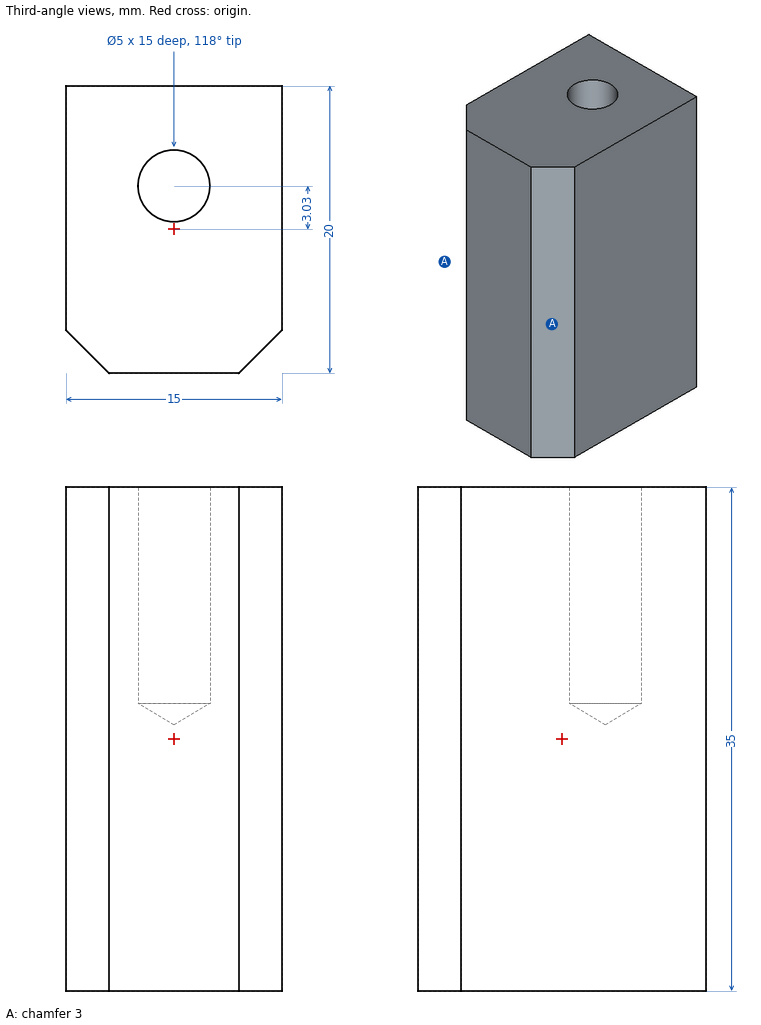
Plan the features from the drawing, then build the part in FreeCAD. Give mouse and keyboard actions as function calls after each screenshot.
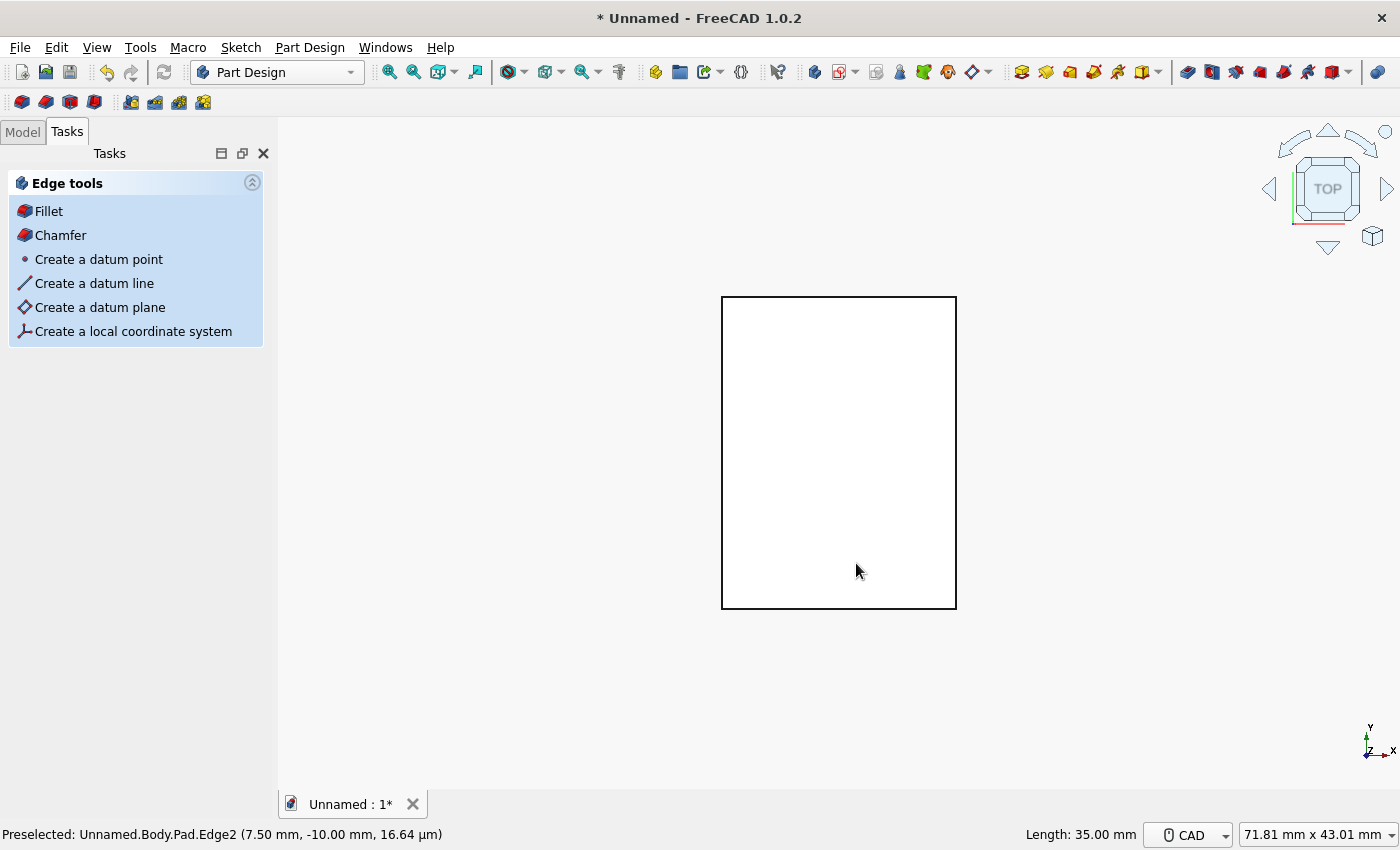
key(1)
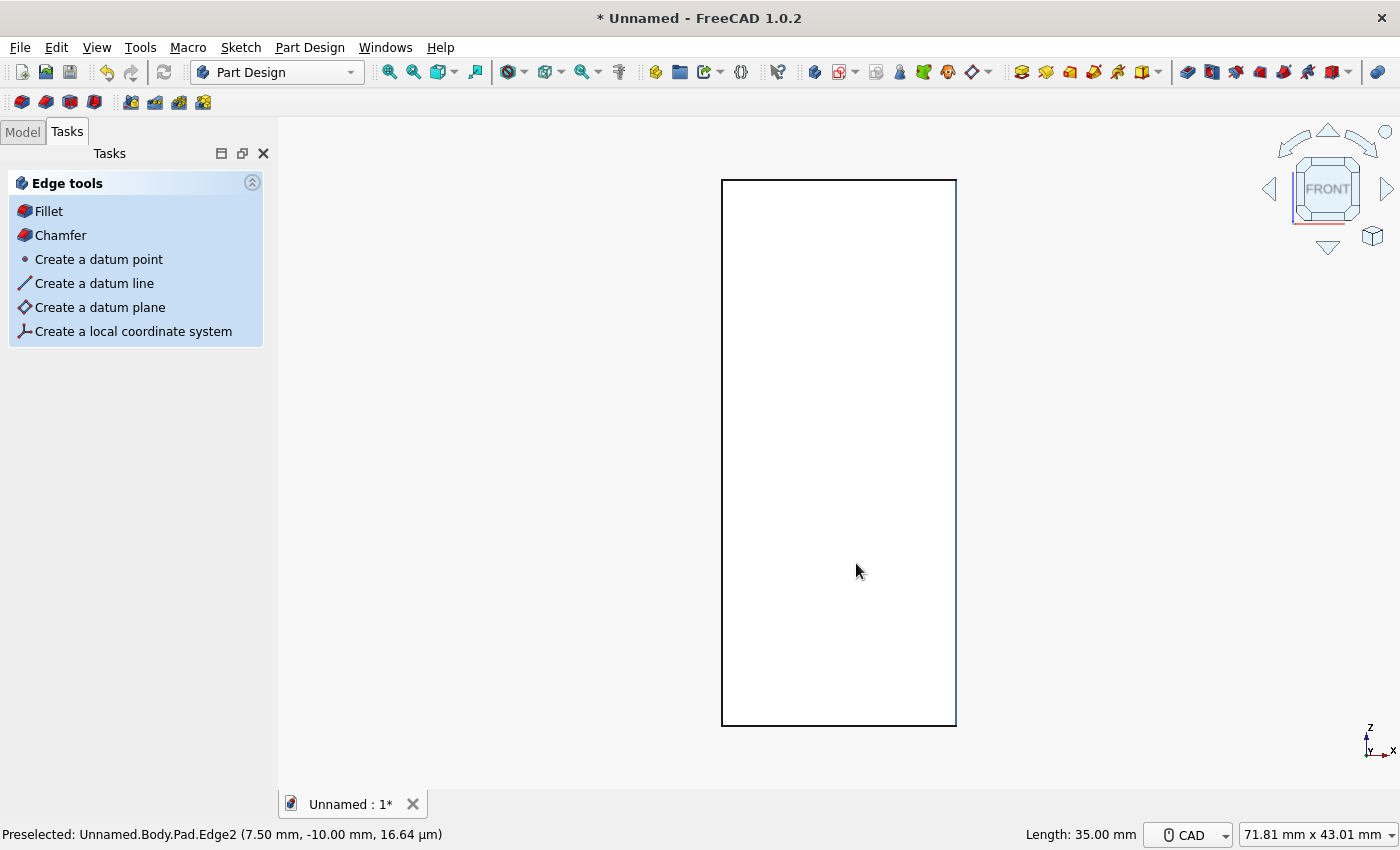
click(722, 452, ctrl)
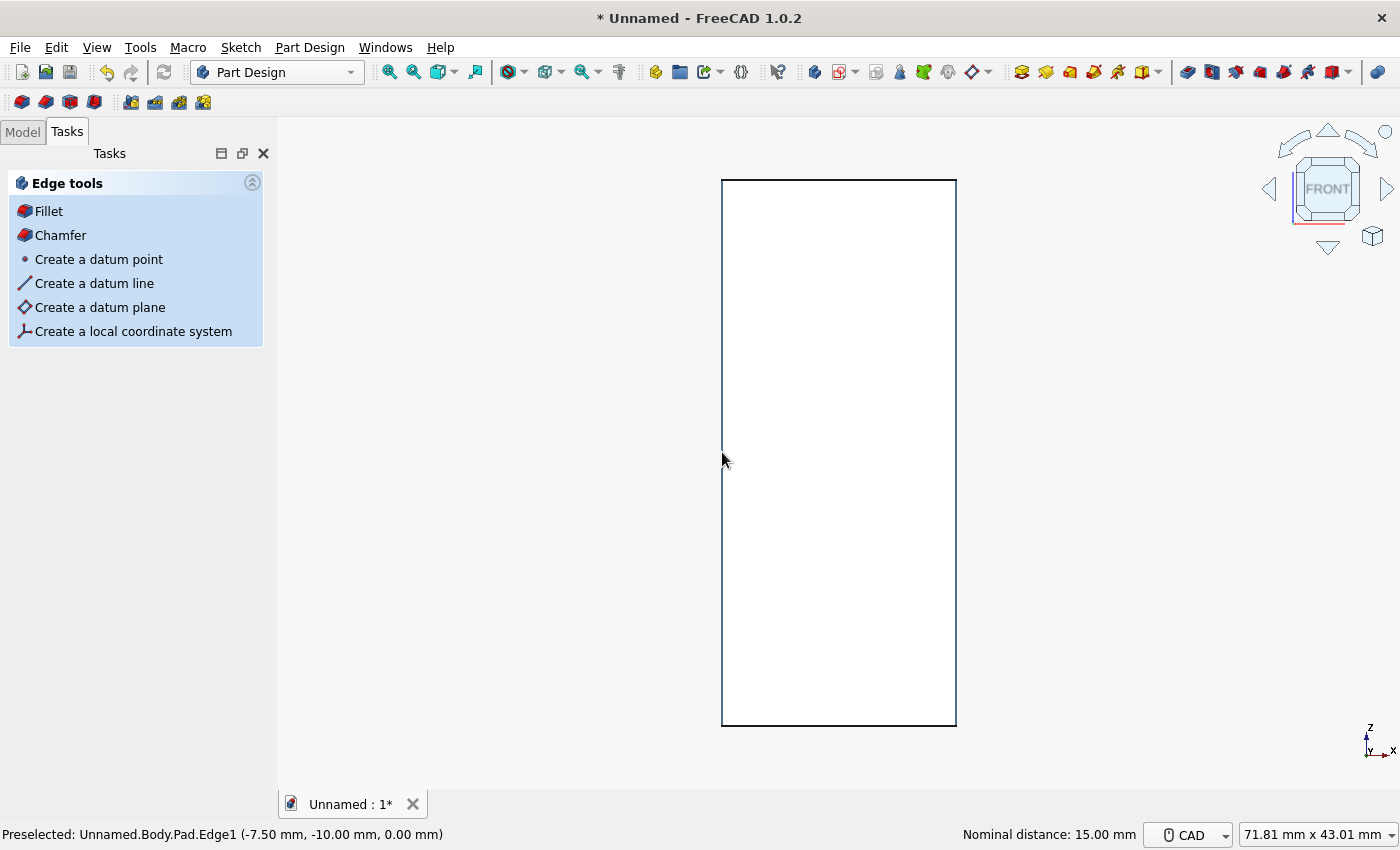
click(46, 102)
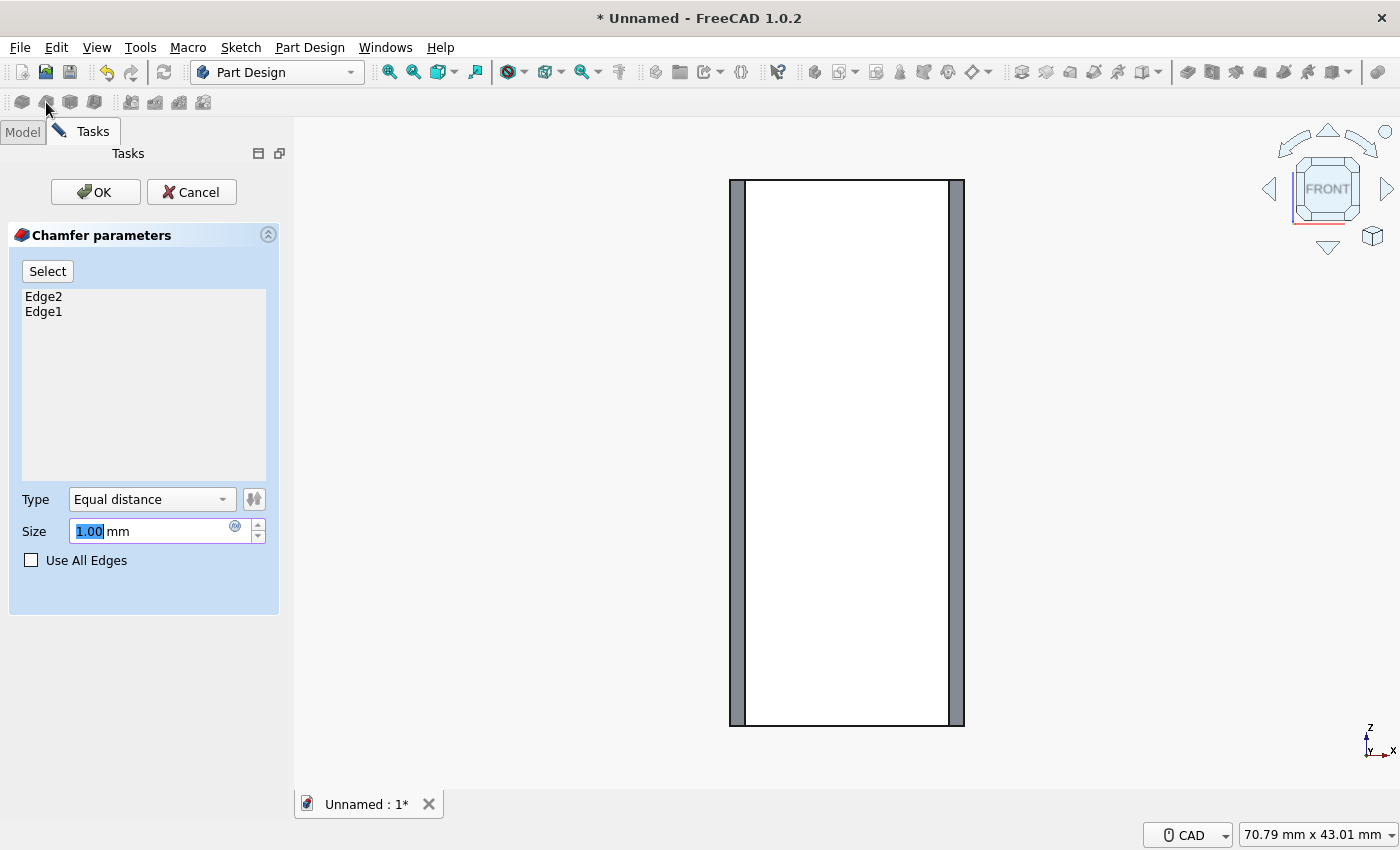
text(3)
key(Tab)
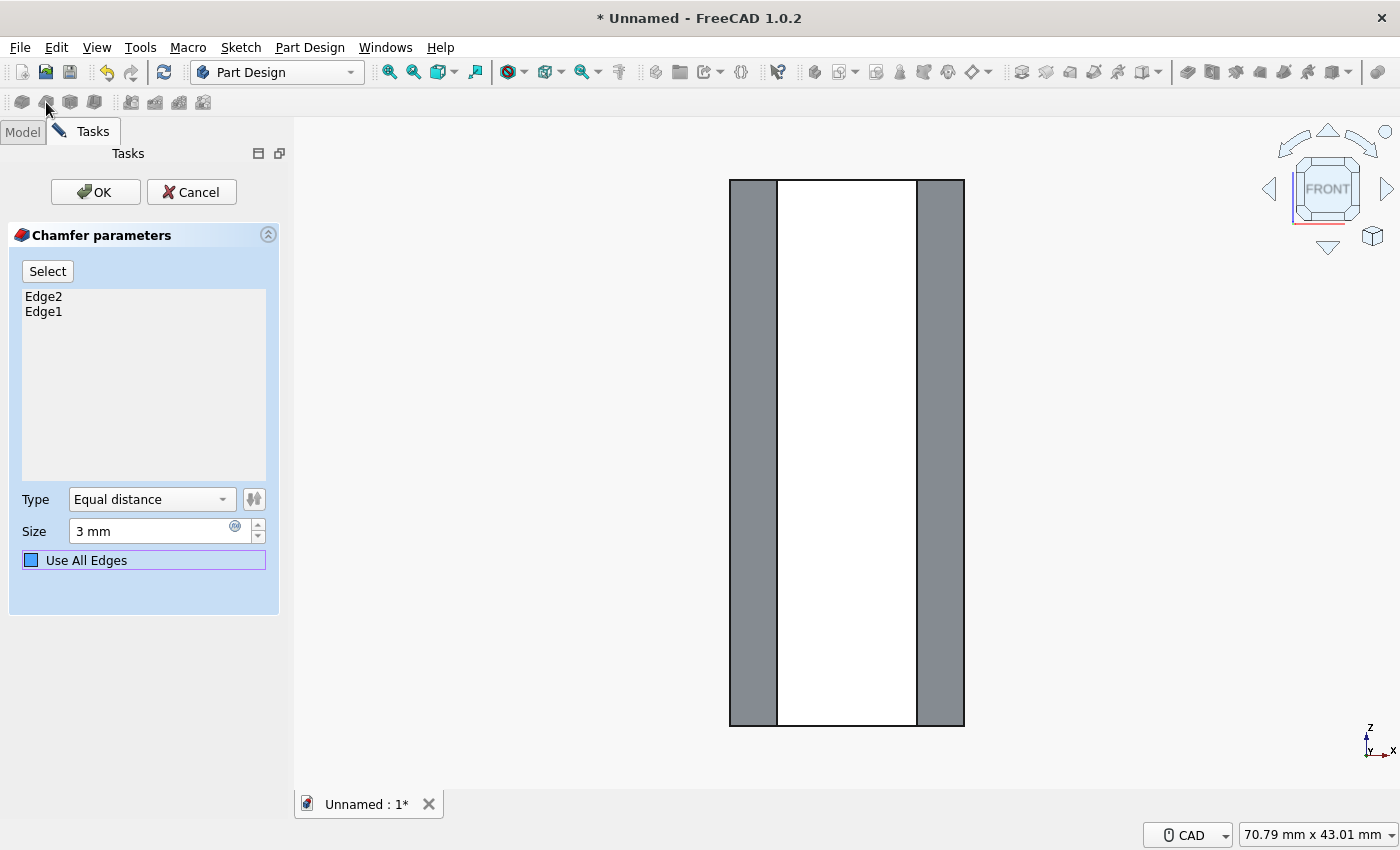
click(96, 192)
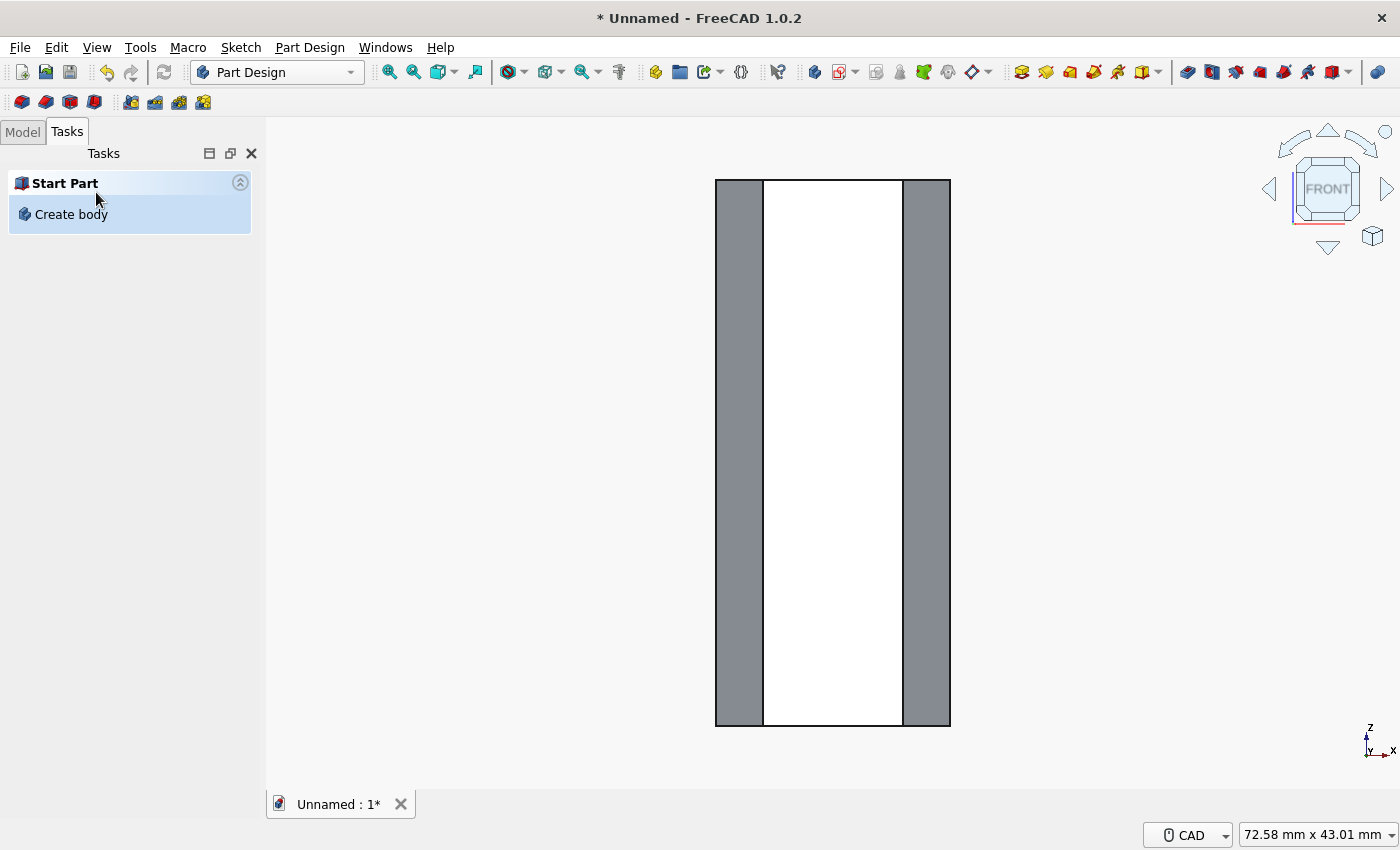
key(0)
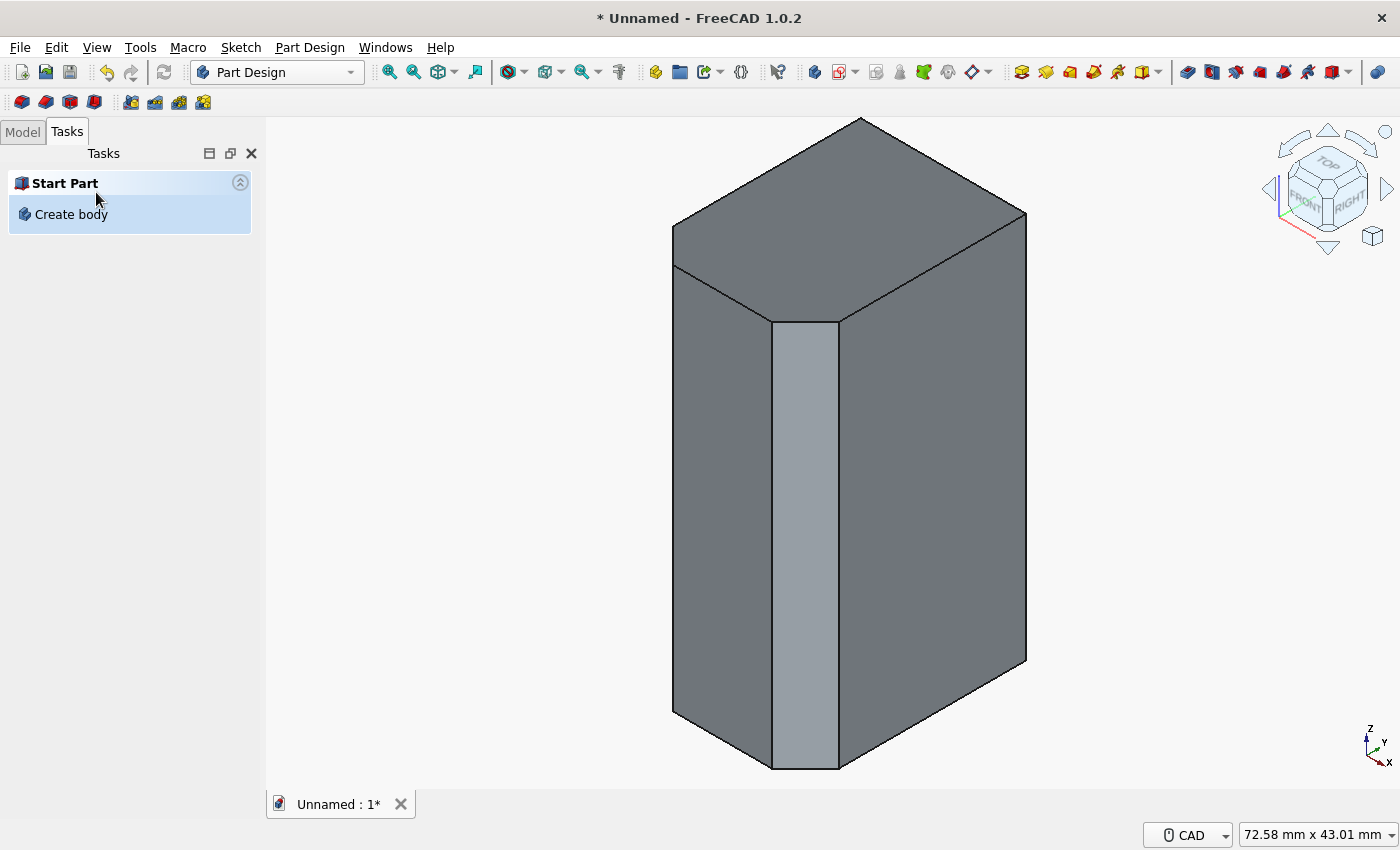
click(833, 229)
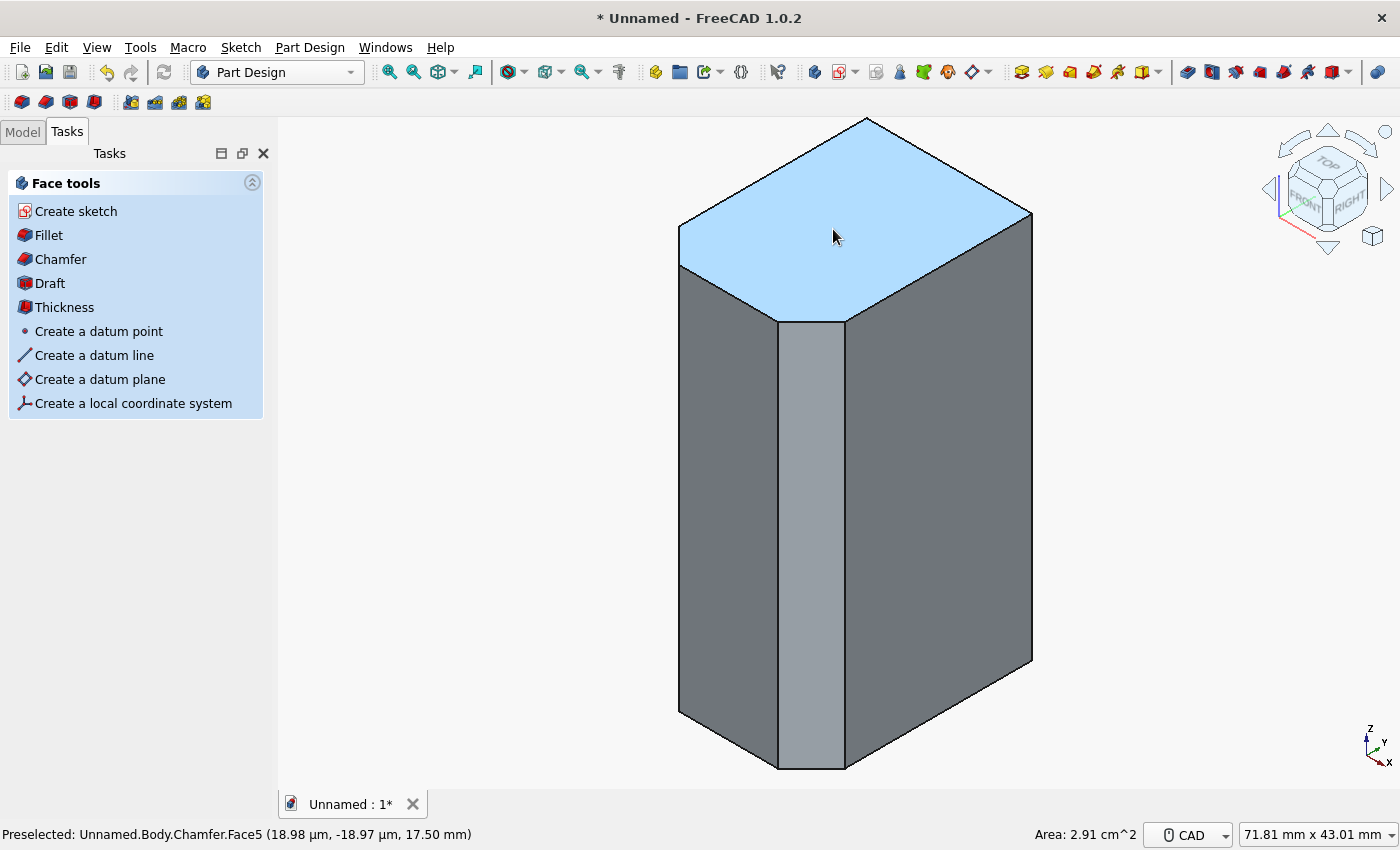
click(840, 72)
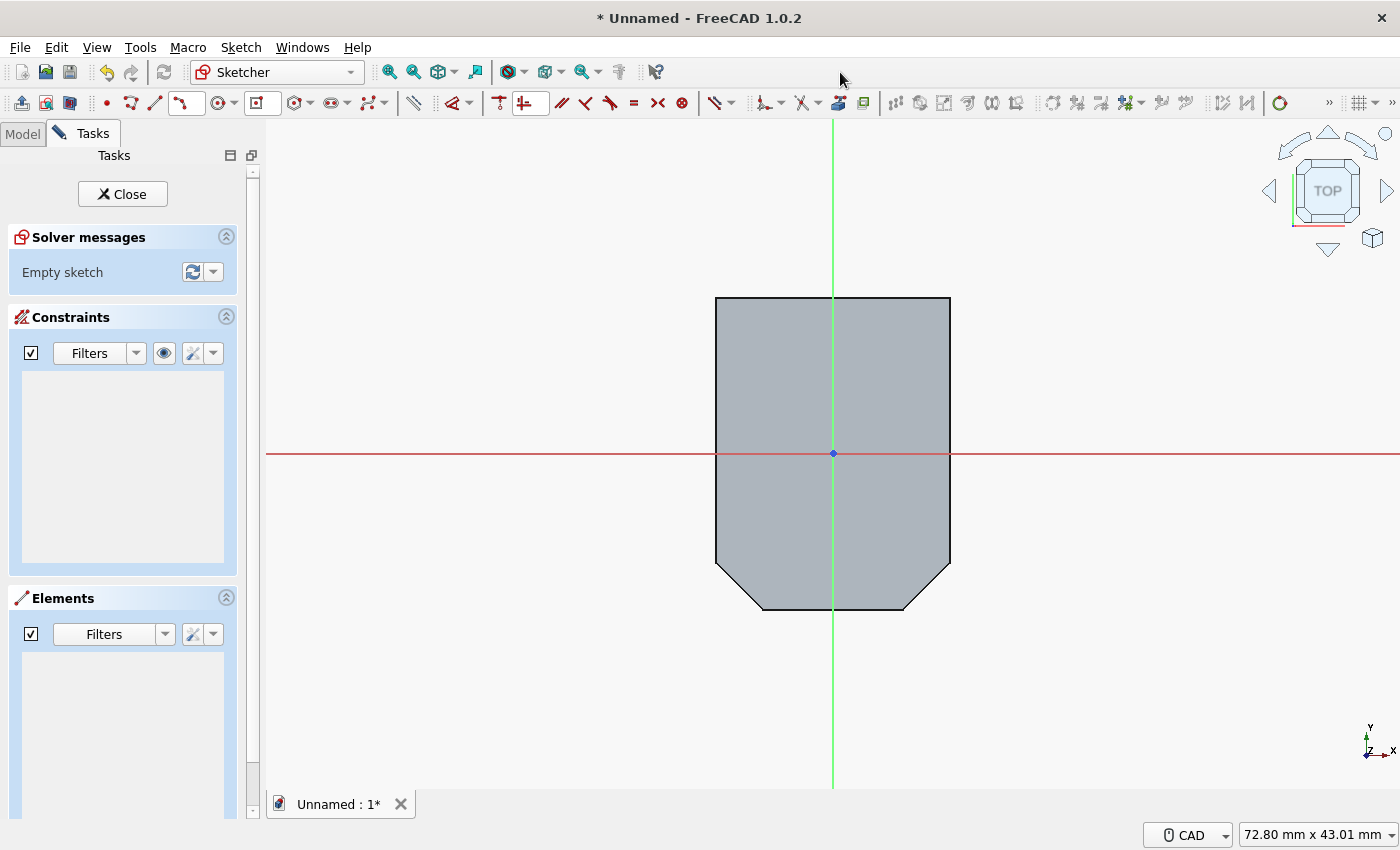
scroll(850, 400, up, 8)